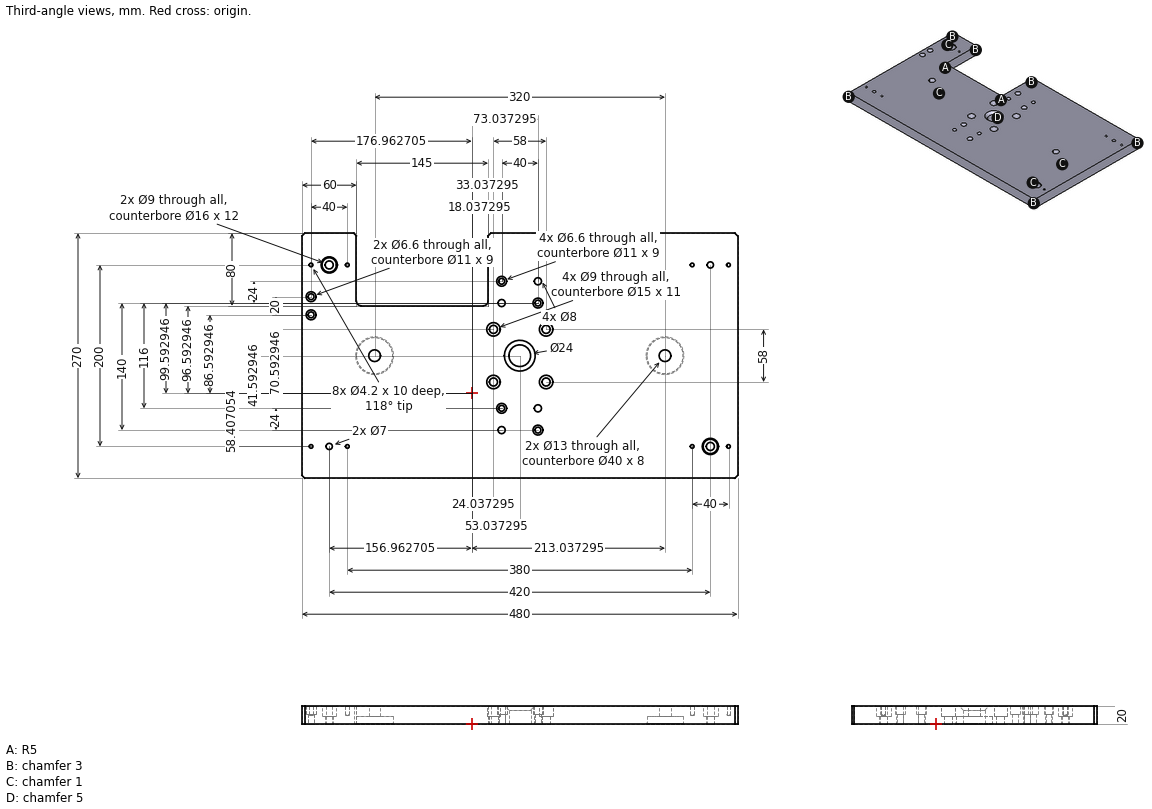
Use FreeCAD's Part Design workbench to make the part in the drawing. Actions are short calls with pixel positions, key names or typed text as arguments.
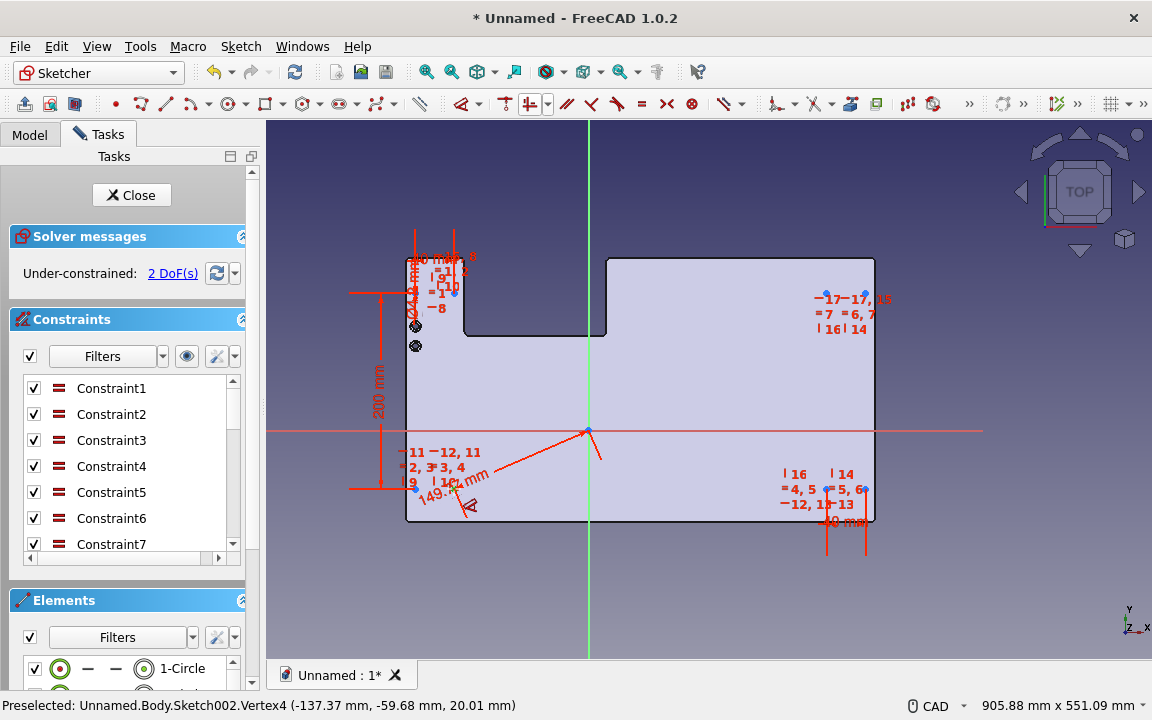
click(827, 489)
click(640, 523)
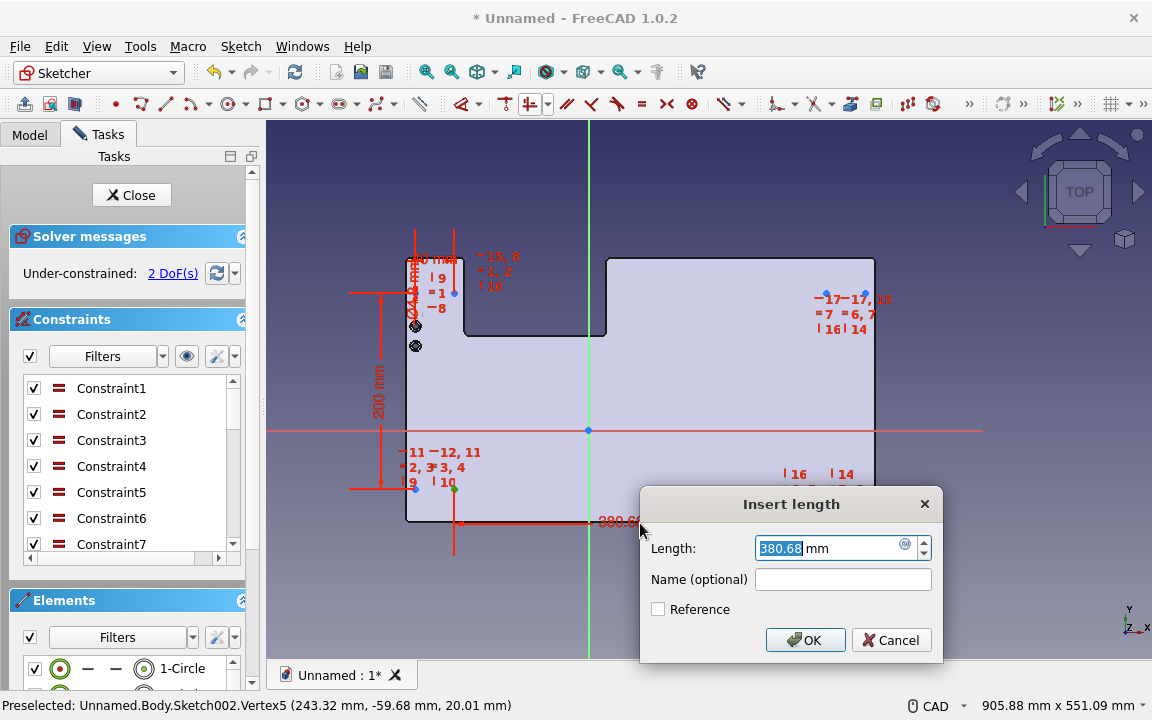
text(380)
key(Return)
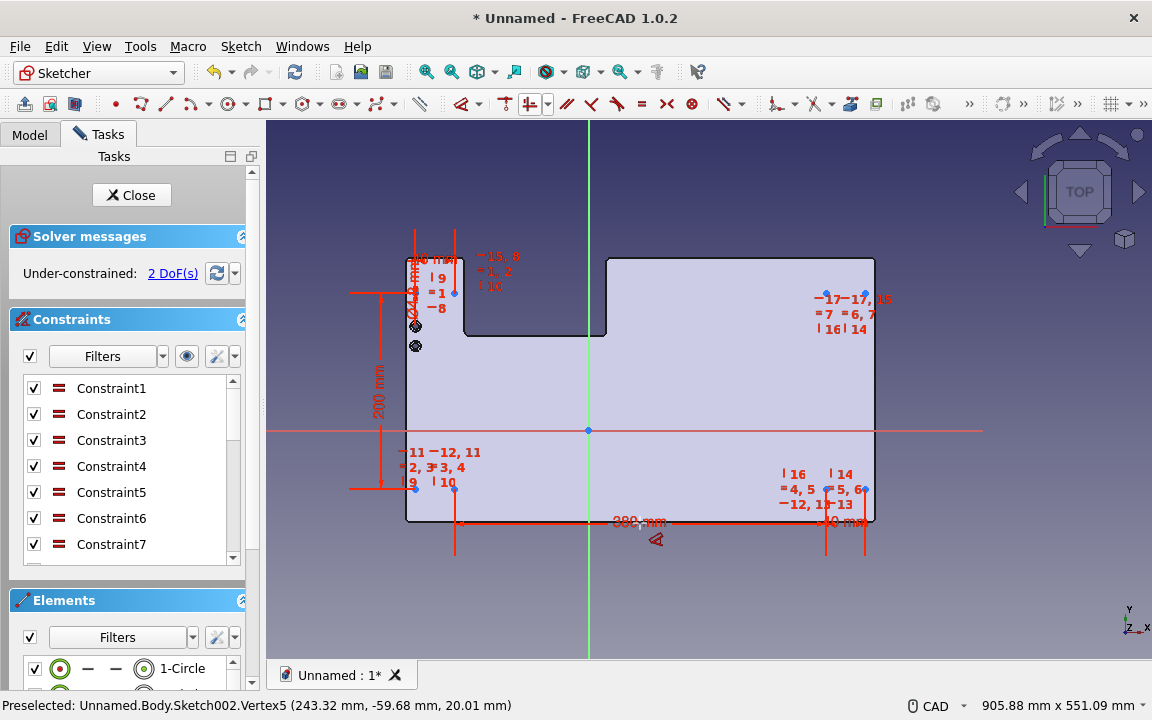
click(415, 489)
click(381, 460)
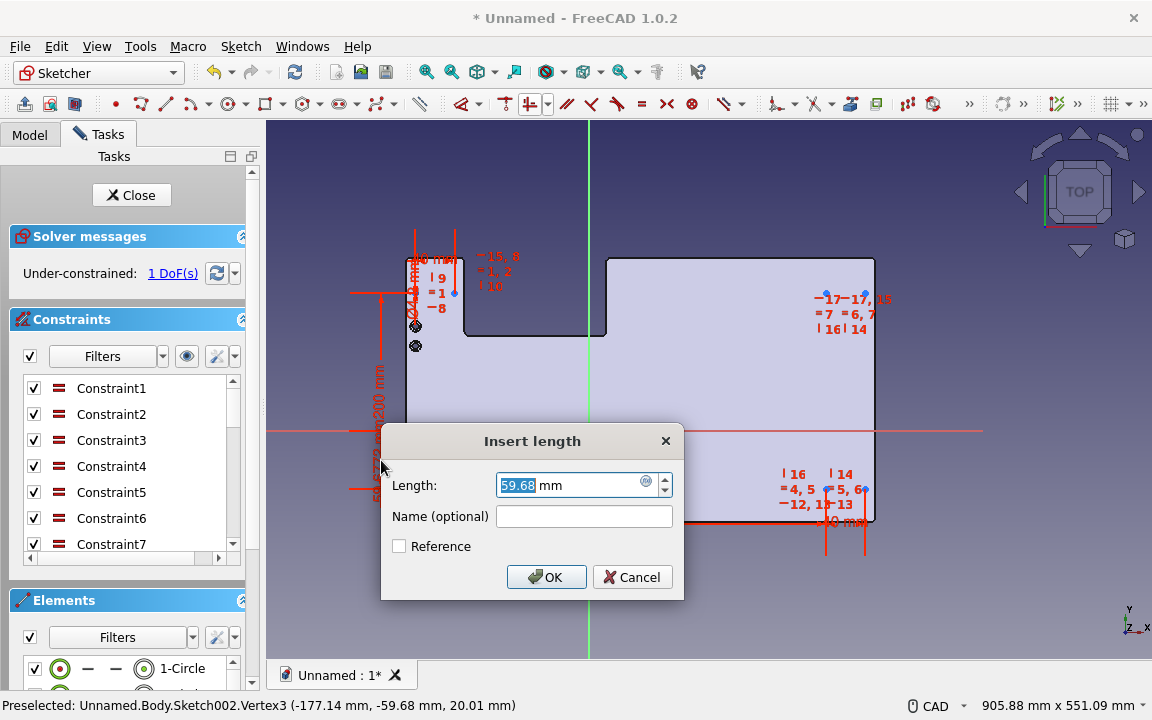
text(58.407054)
key(Return)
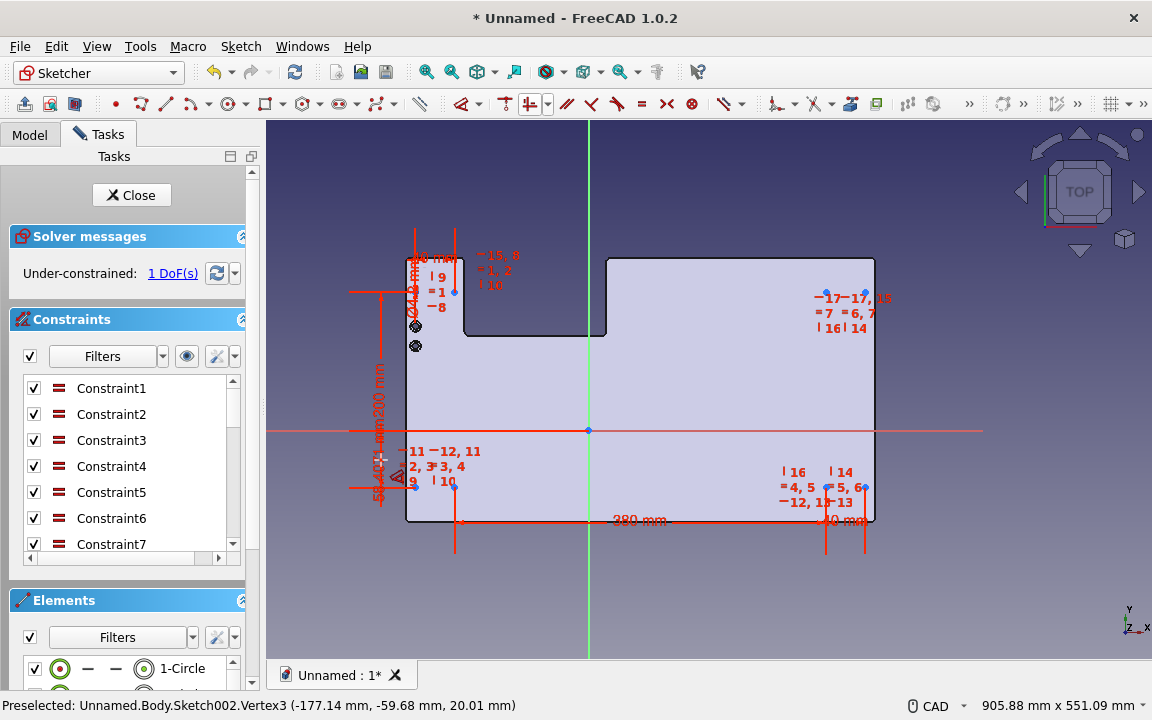
click(415, 292)
click(542, 258)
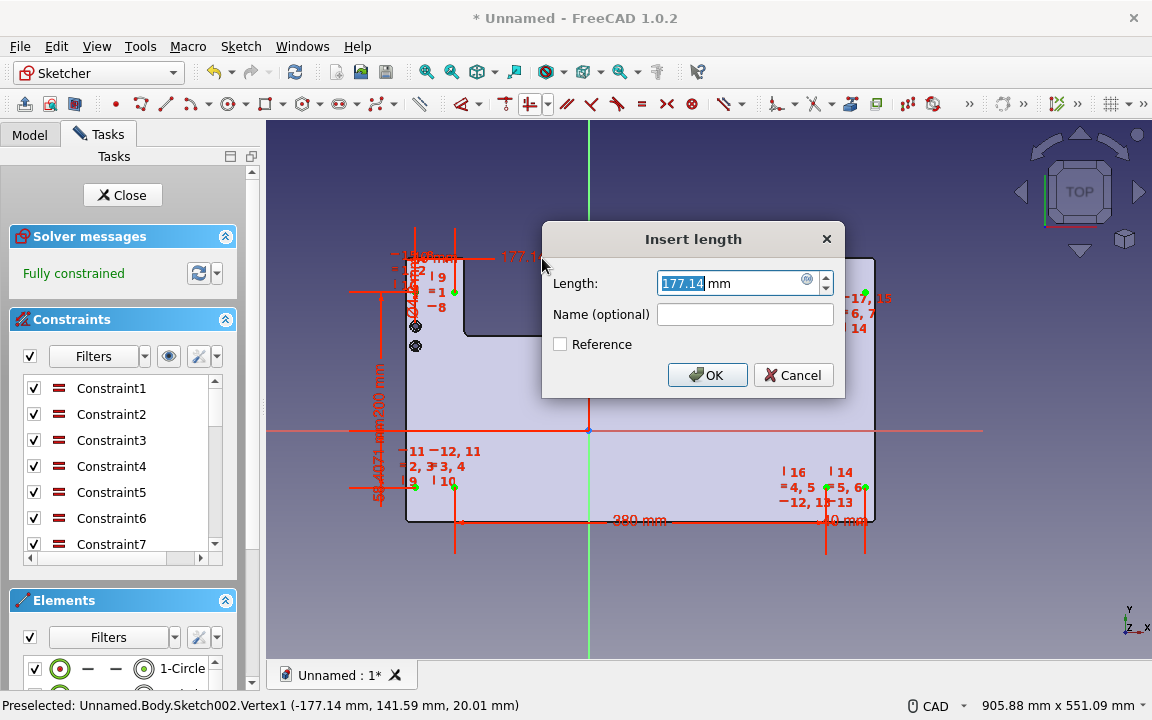
text(176.962705)
key(Return)
key(Escape)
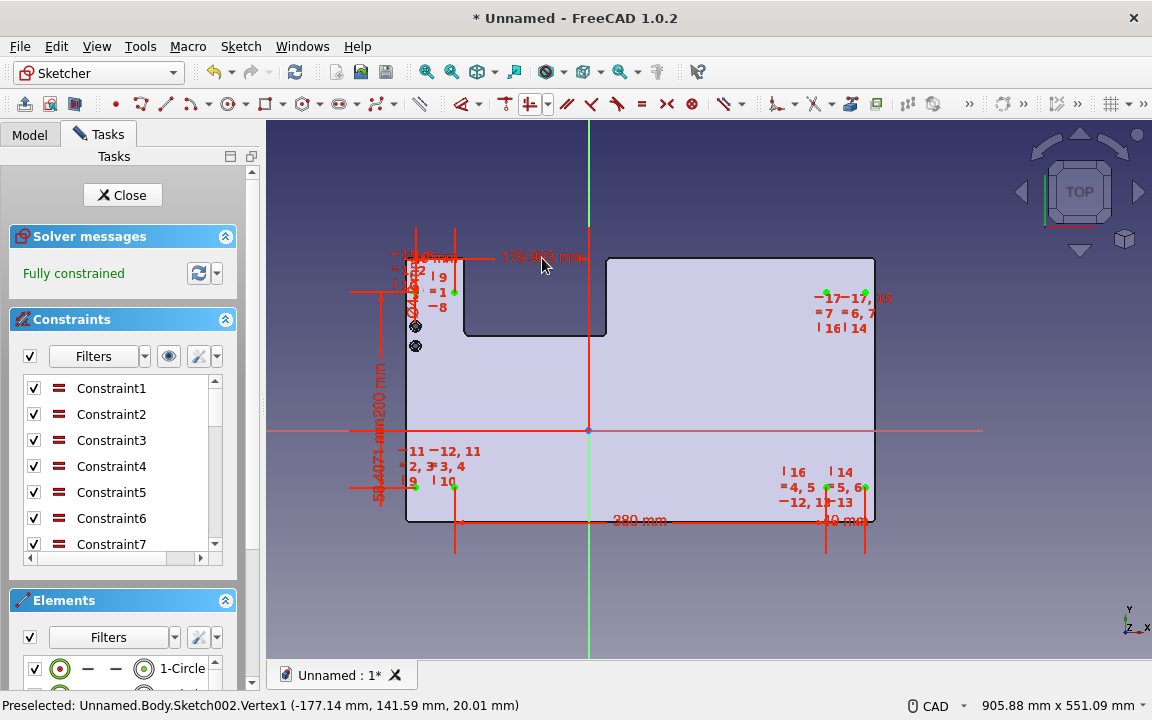
click(123, 195)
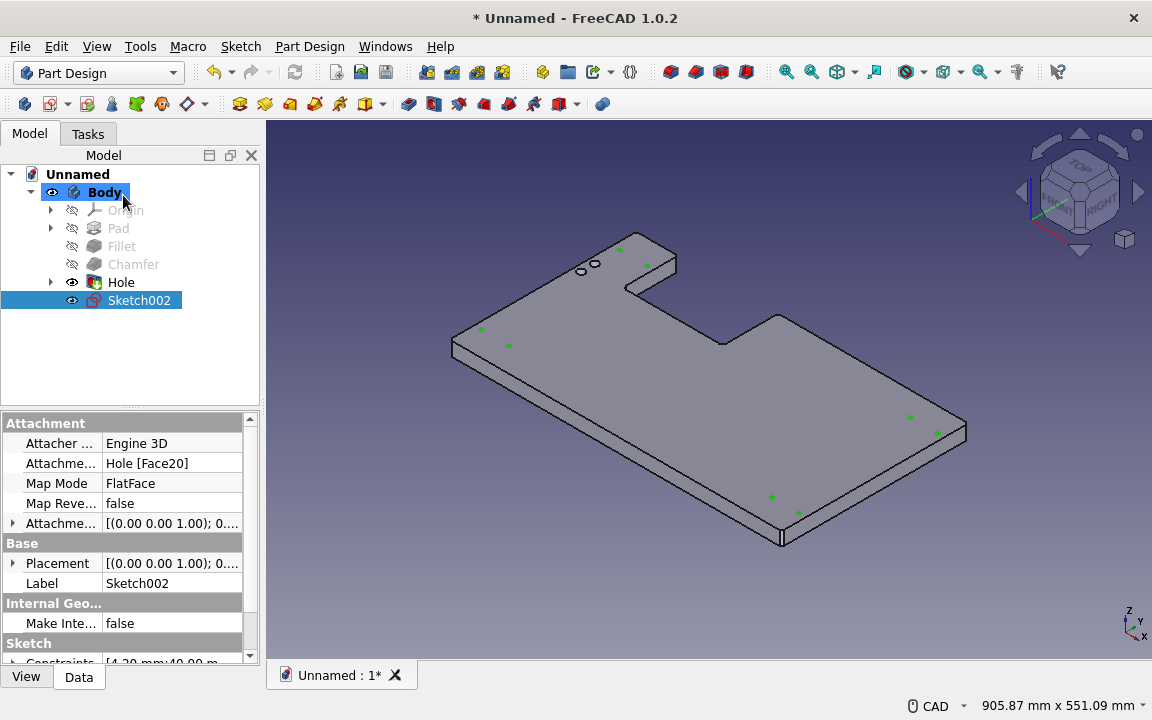
click(434, 104)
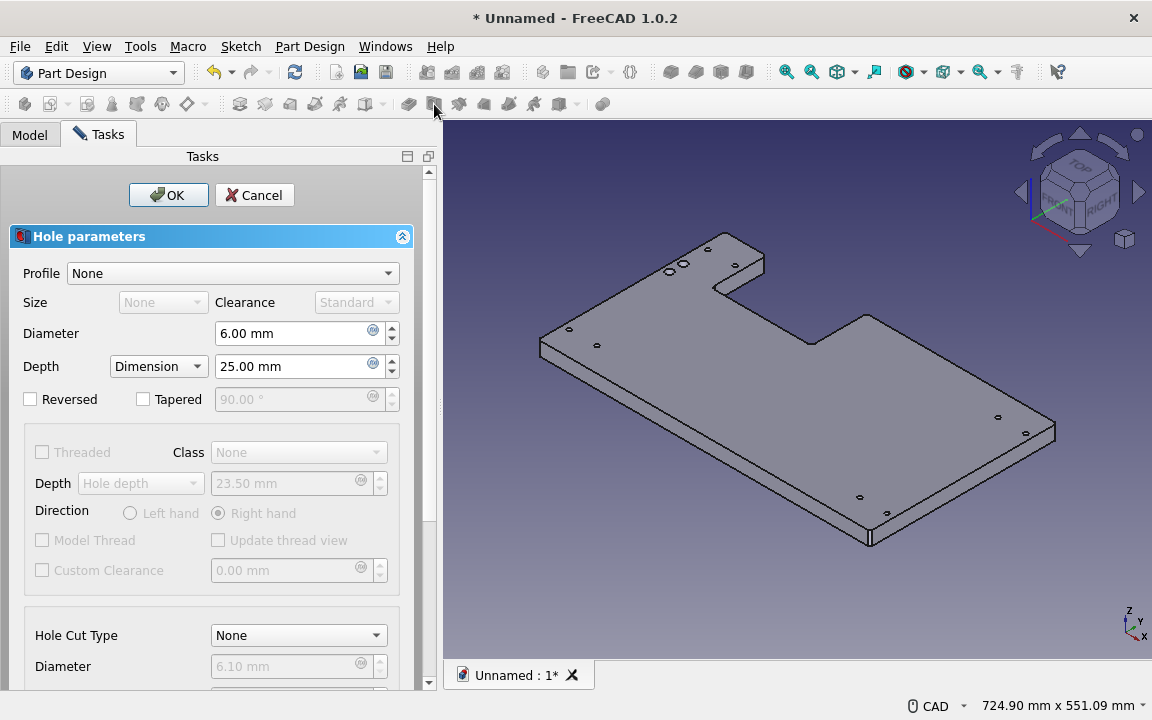
triple_click(300, 334)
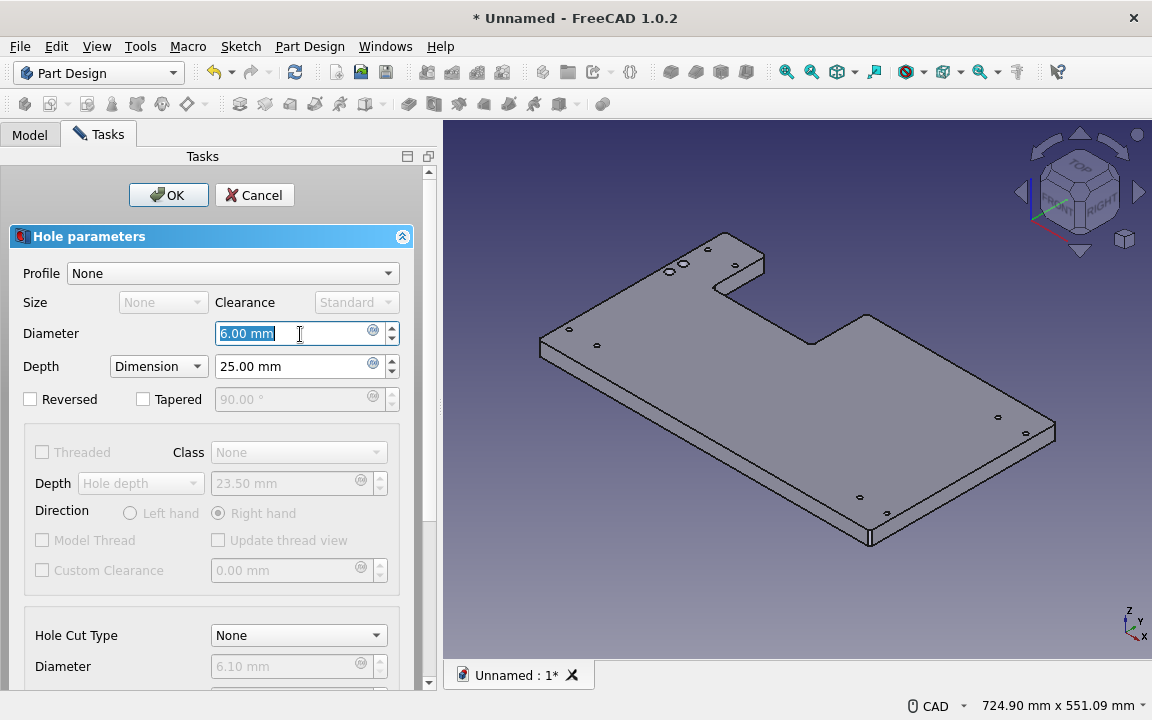
text(4.2)
key(Tab)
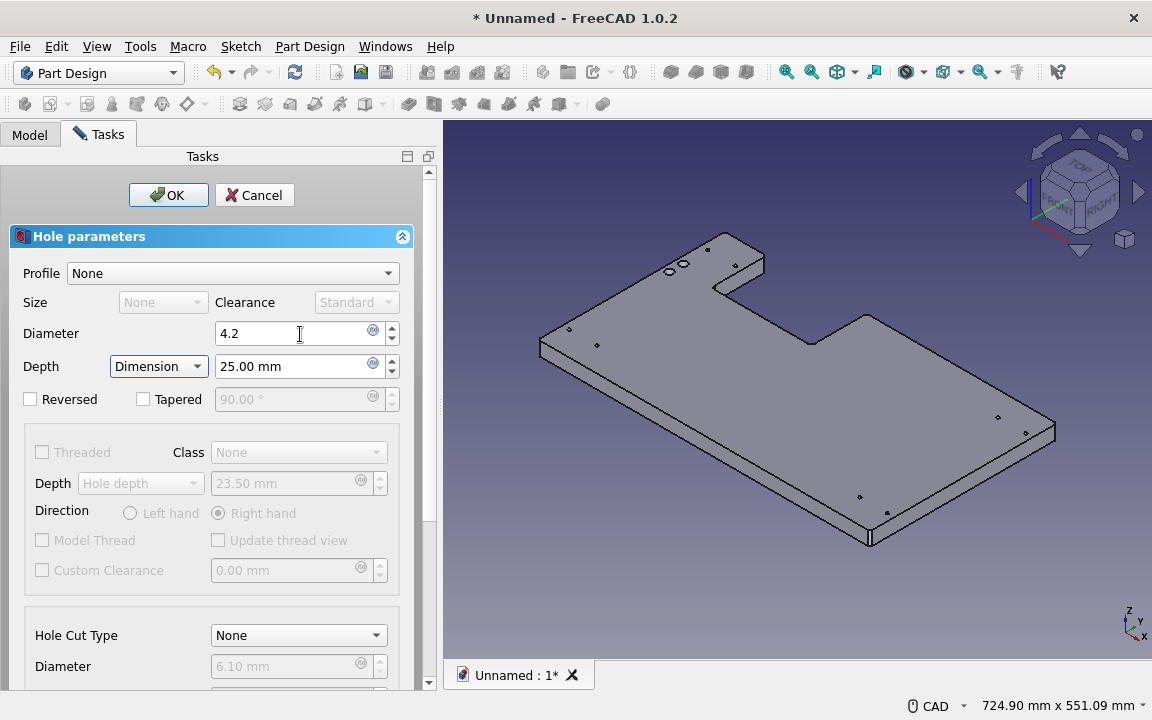
triple_click(300, 366)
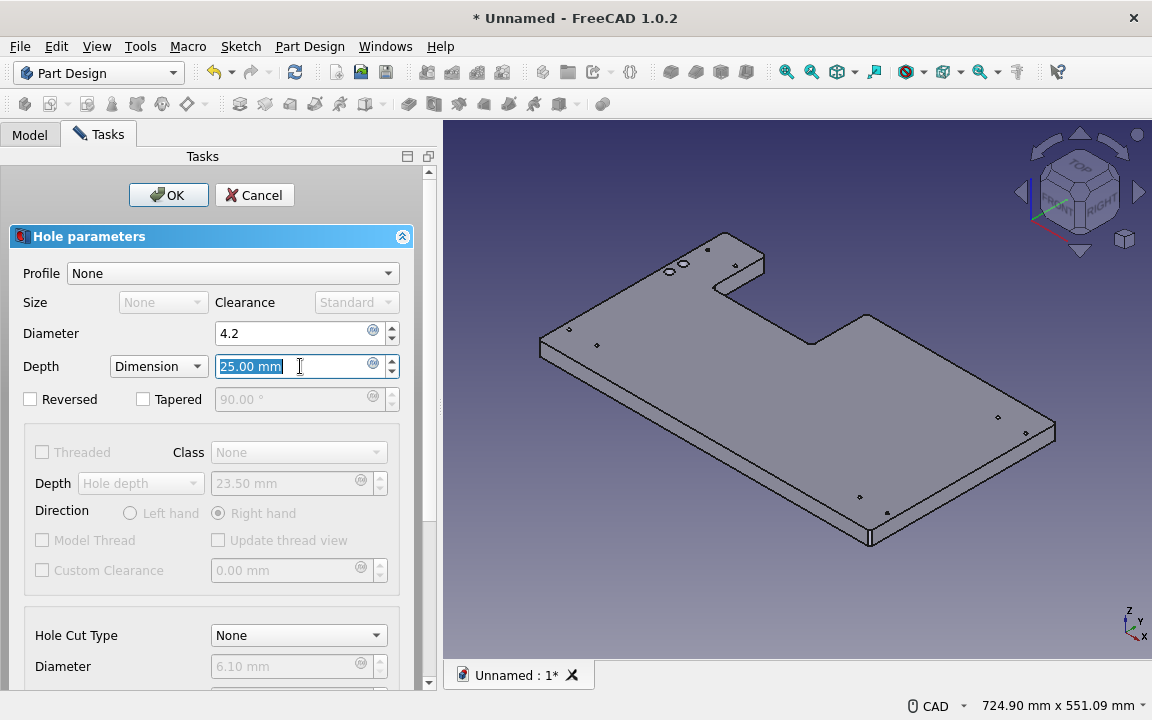
text(10)
key(Tab)